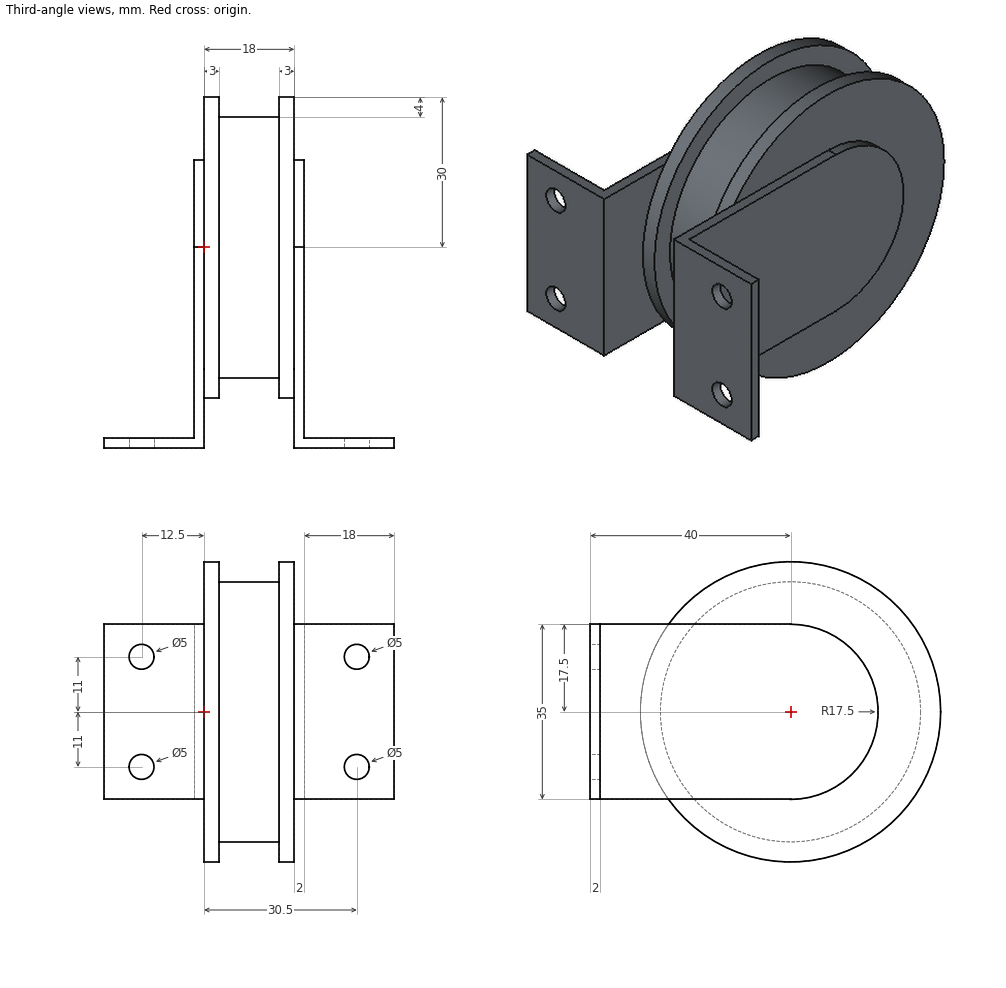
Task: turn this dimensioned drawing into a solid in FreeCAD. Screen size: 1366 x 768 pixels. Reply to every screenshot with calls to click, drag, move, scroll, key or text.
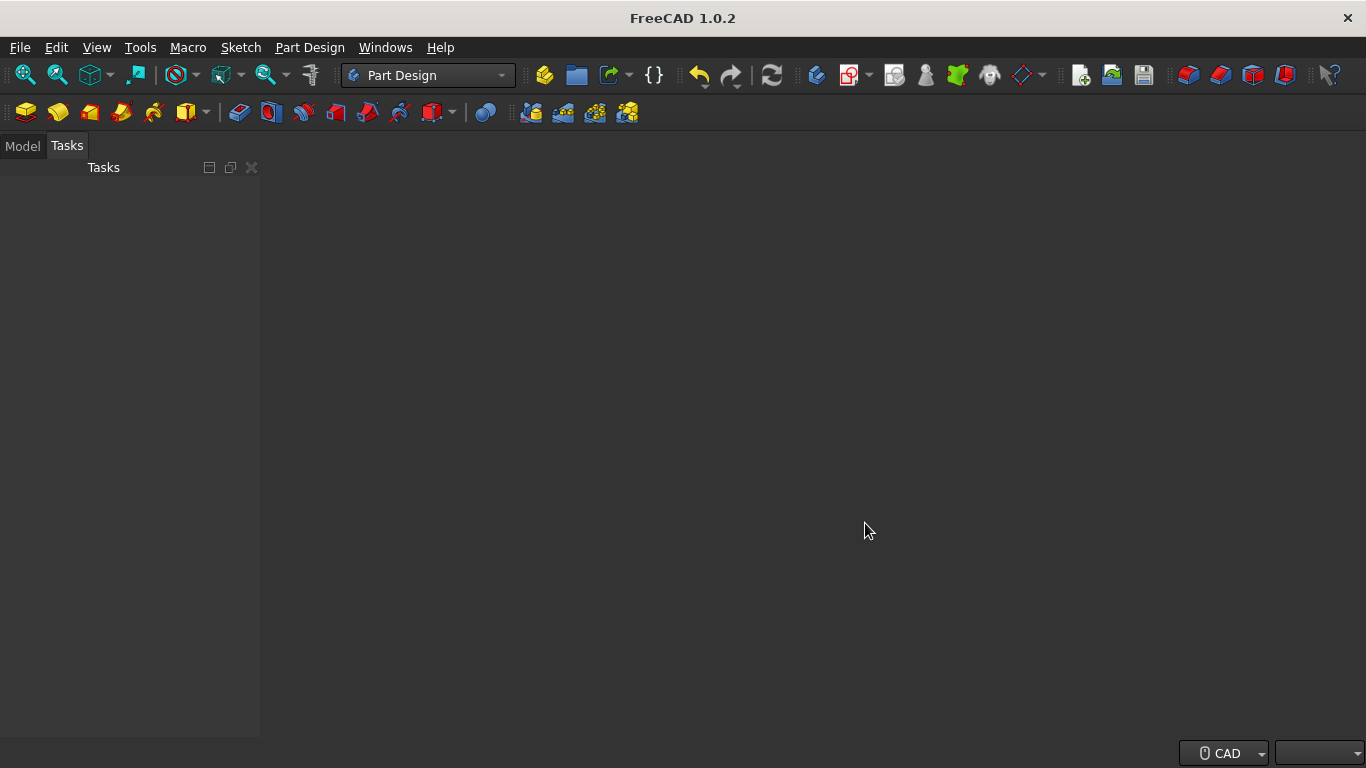
click(1080, 76)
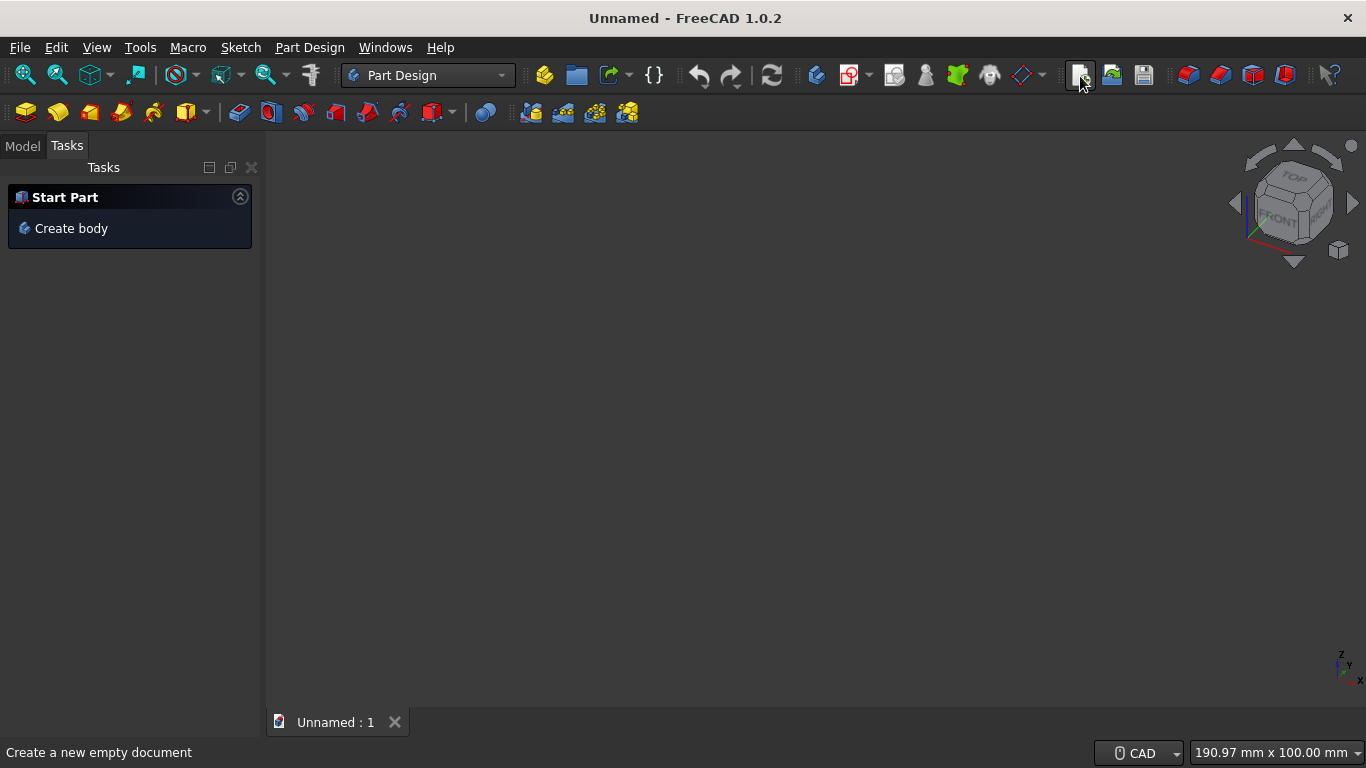
click(850, 76)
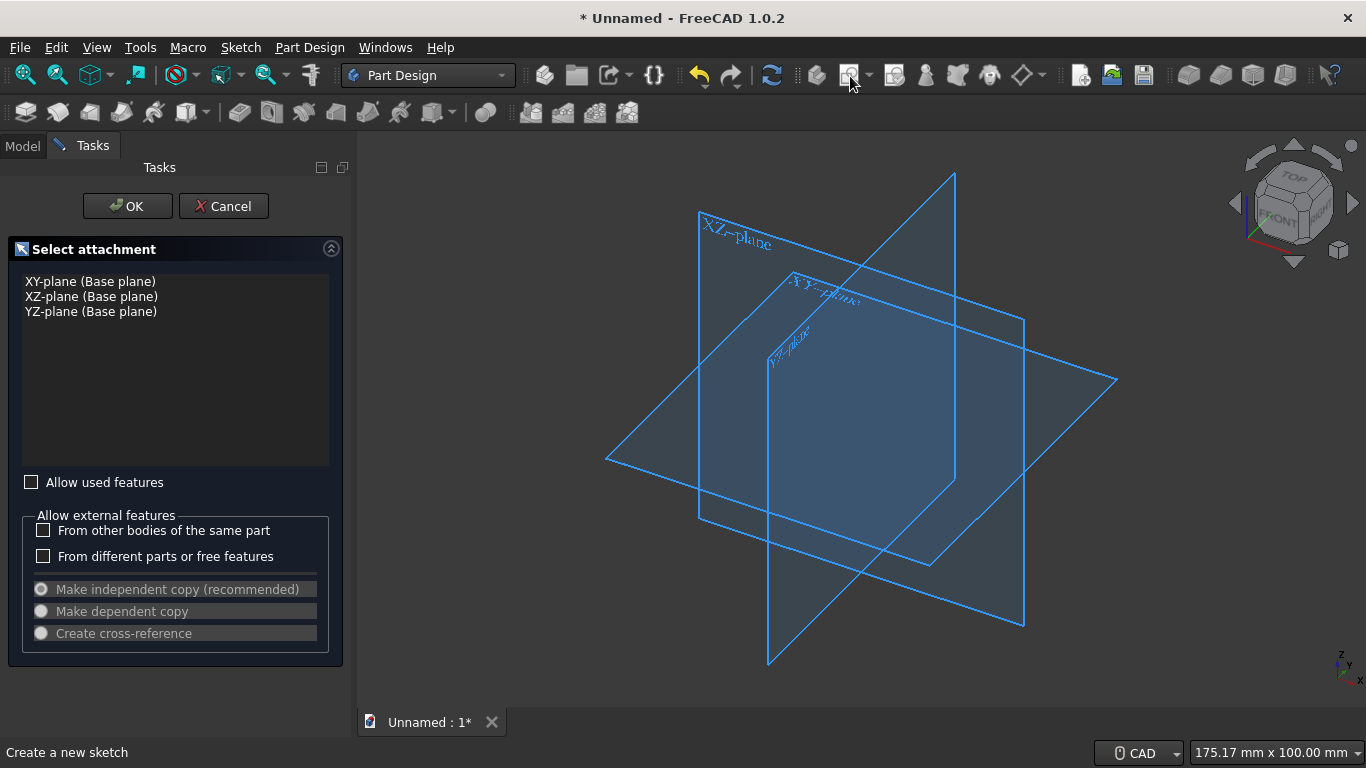
click(82, 282)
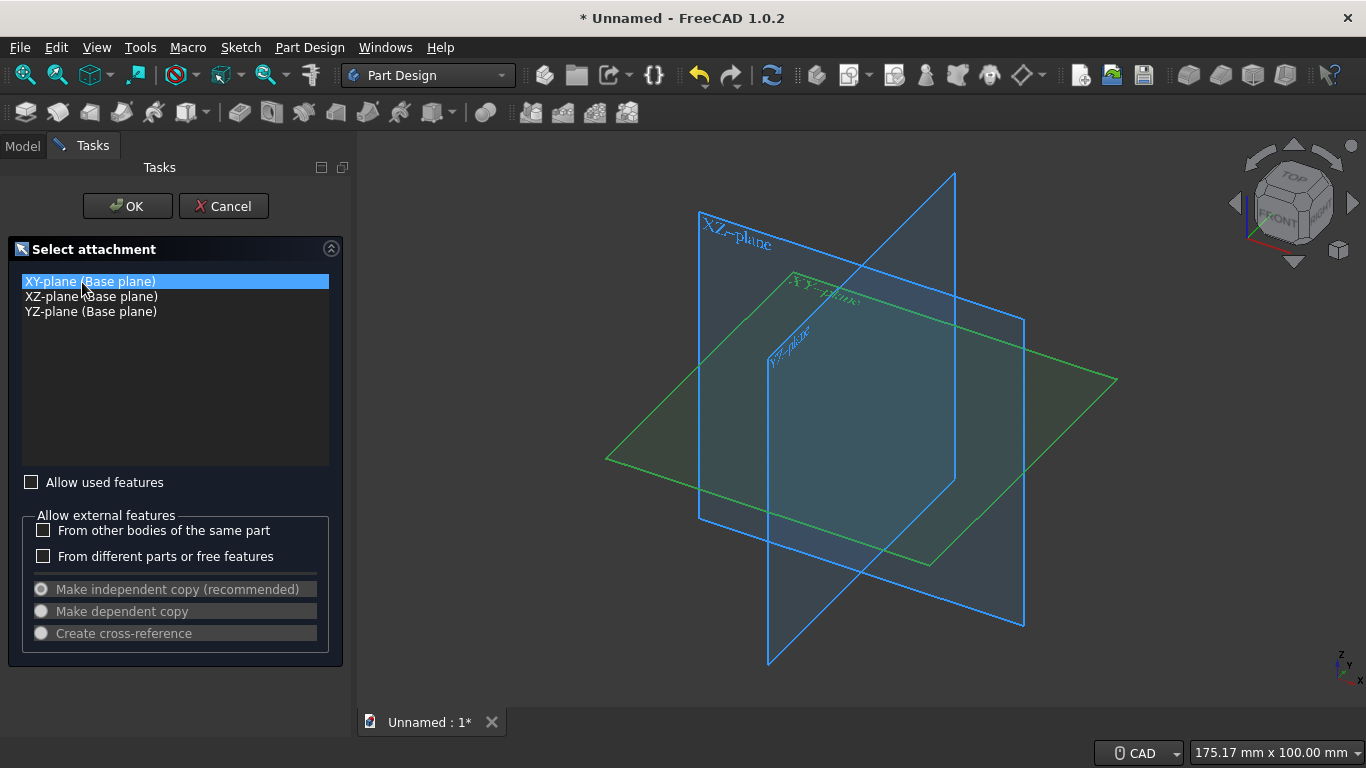
click(128, 206)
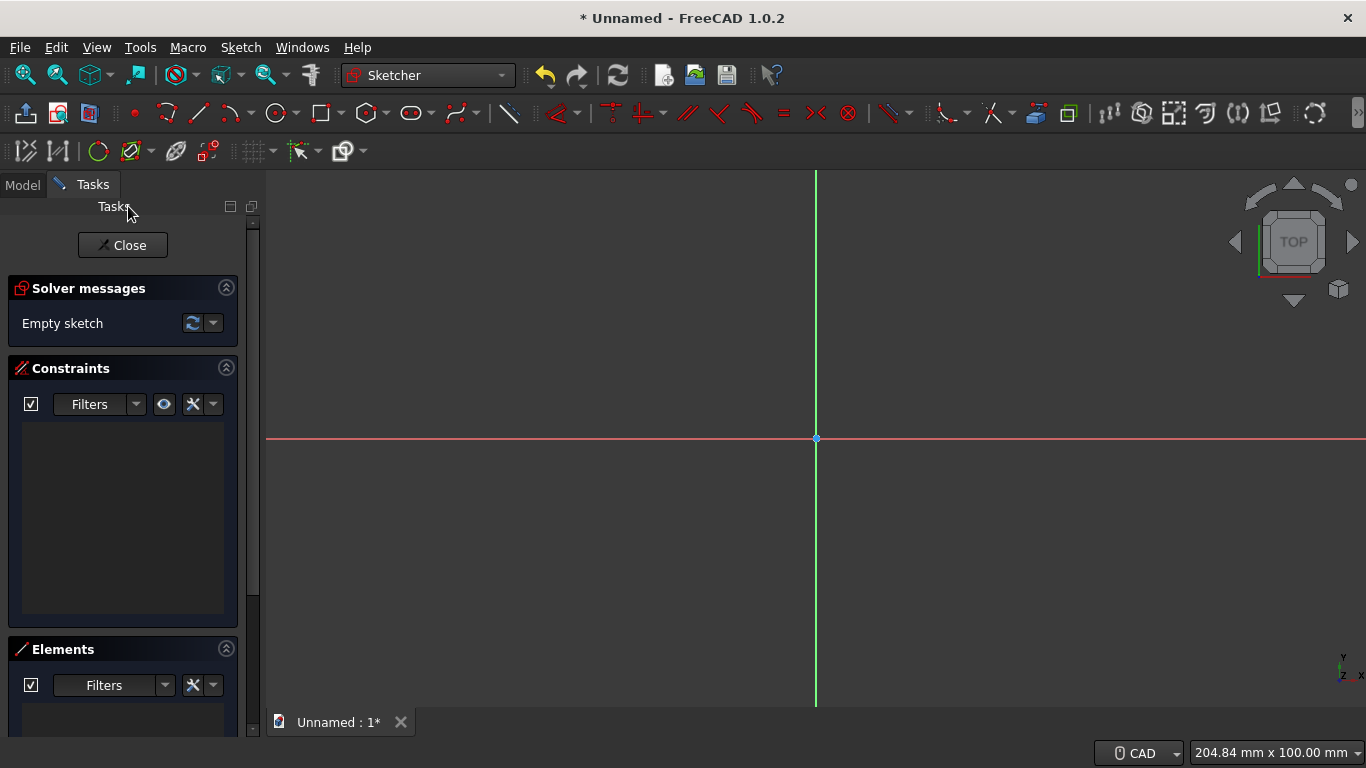
scroll(960, 292, up, 4)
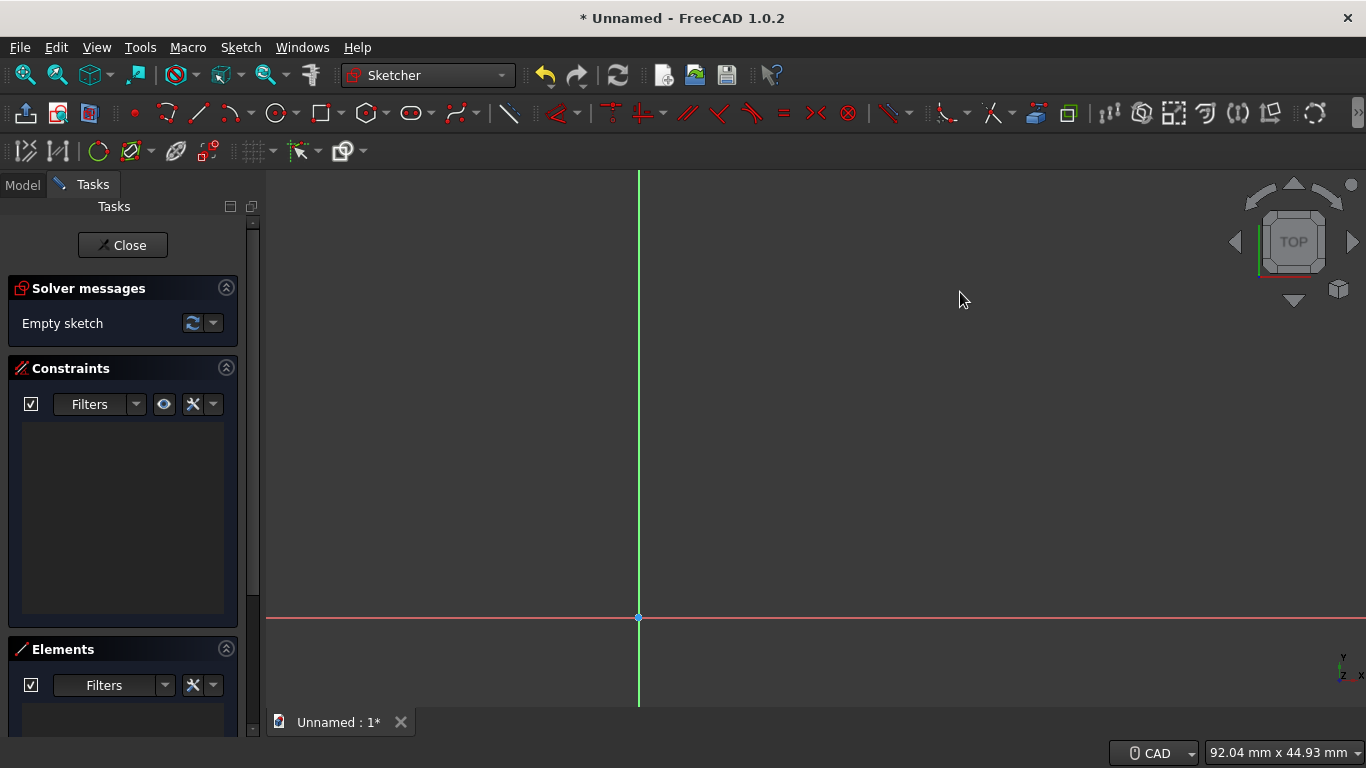
key(g)
key(m)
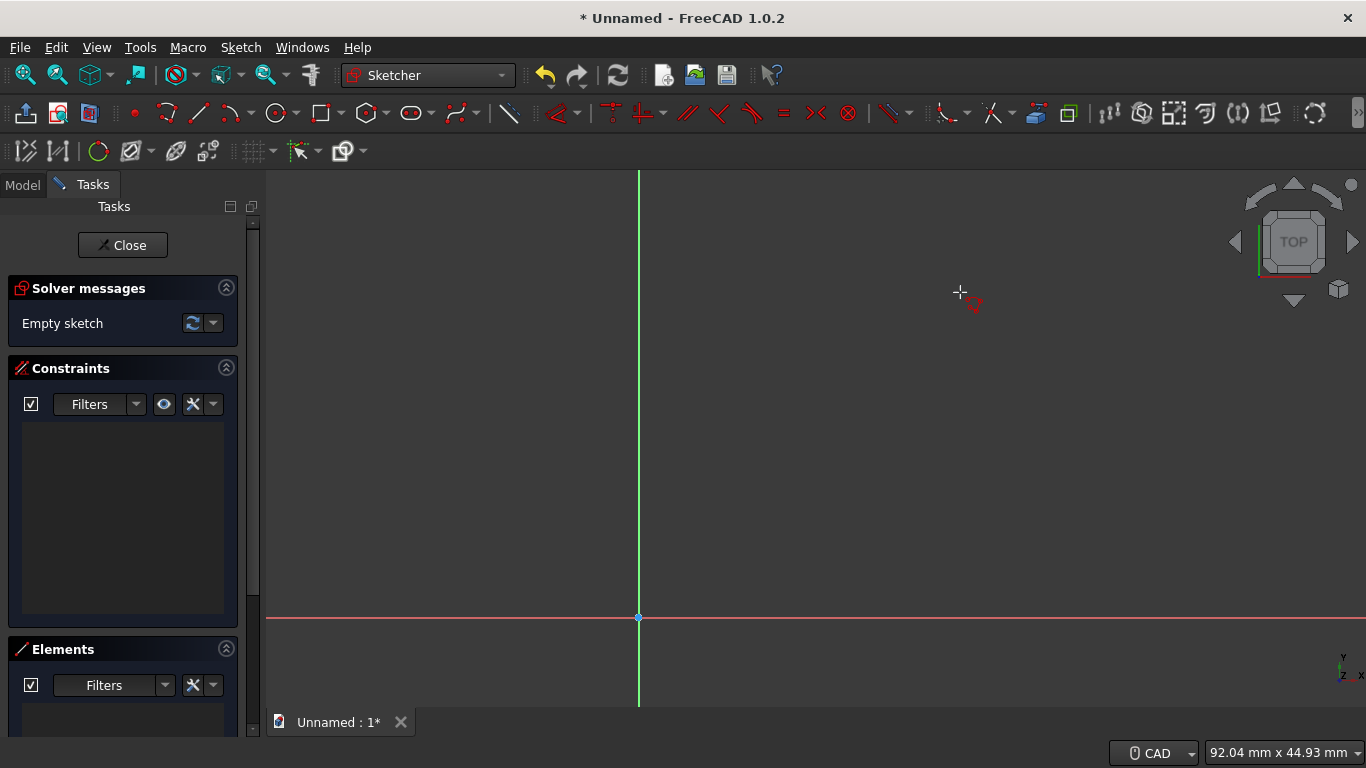
click(639, 618)
click(854, 609)
click(854, 259)
click(818, 259)
click(818, 307)
click(675, 307)
click(675, 259)
click(648, 259)
click(639, 618)
key(Escape)
key(Escape)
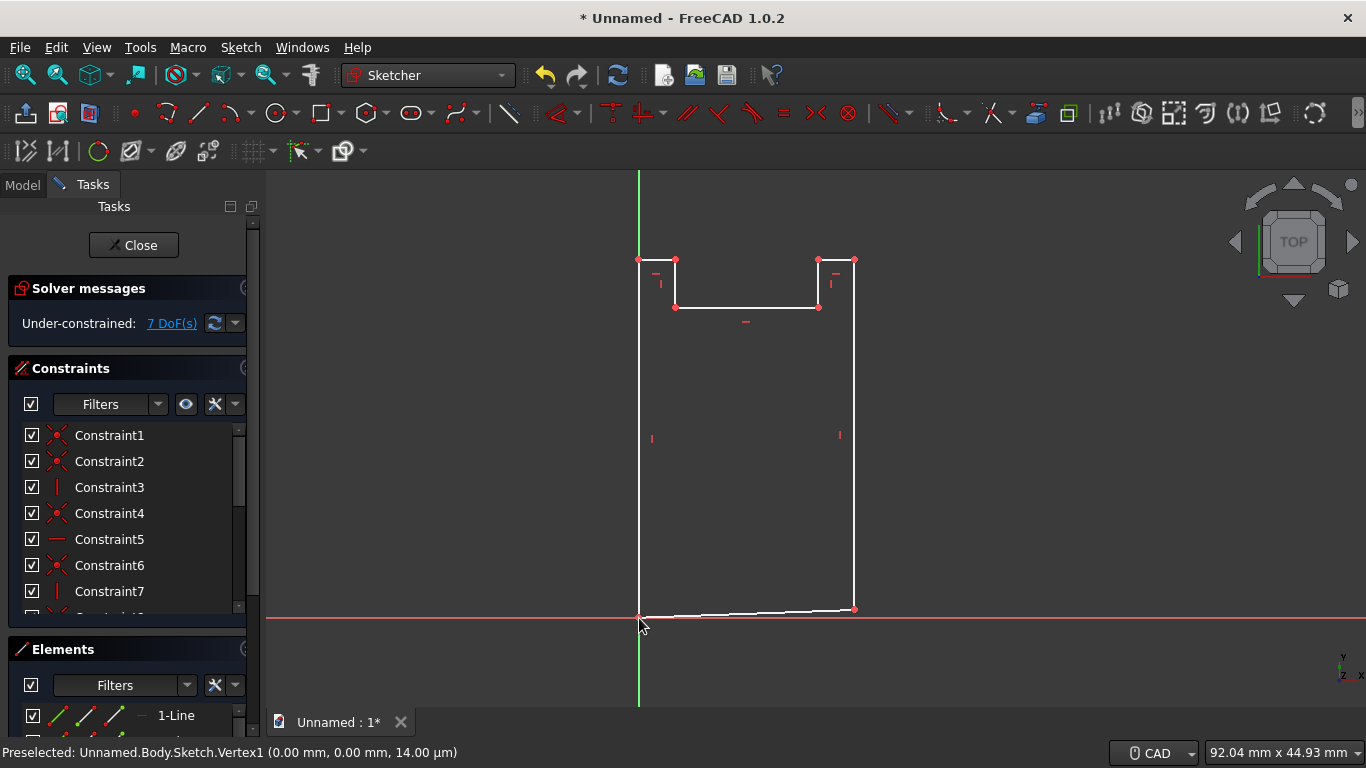
click(703, 615)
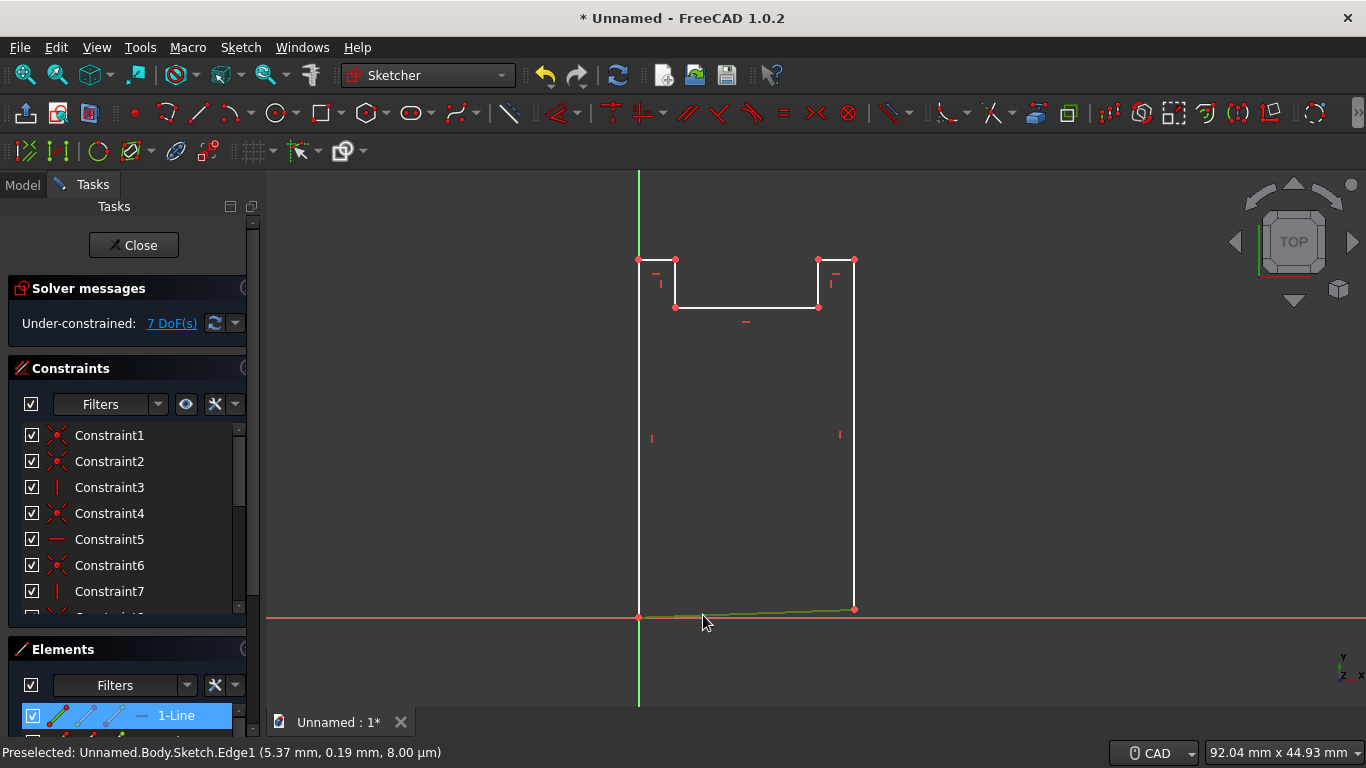
click(666, 114)